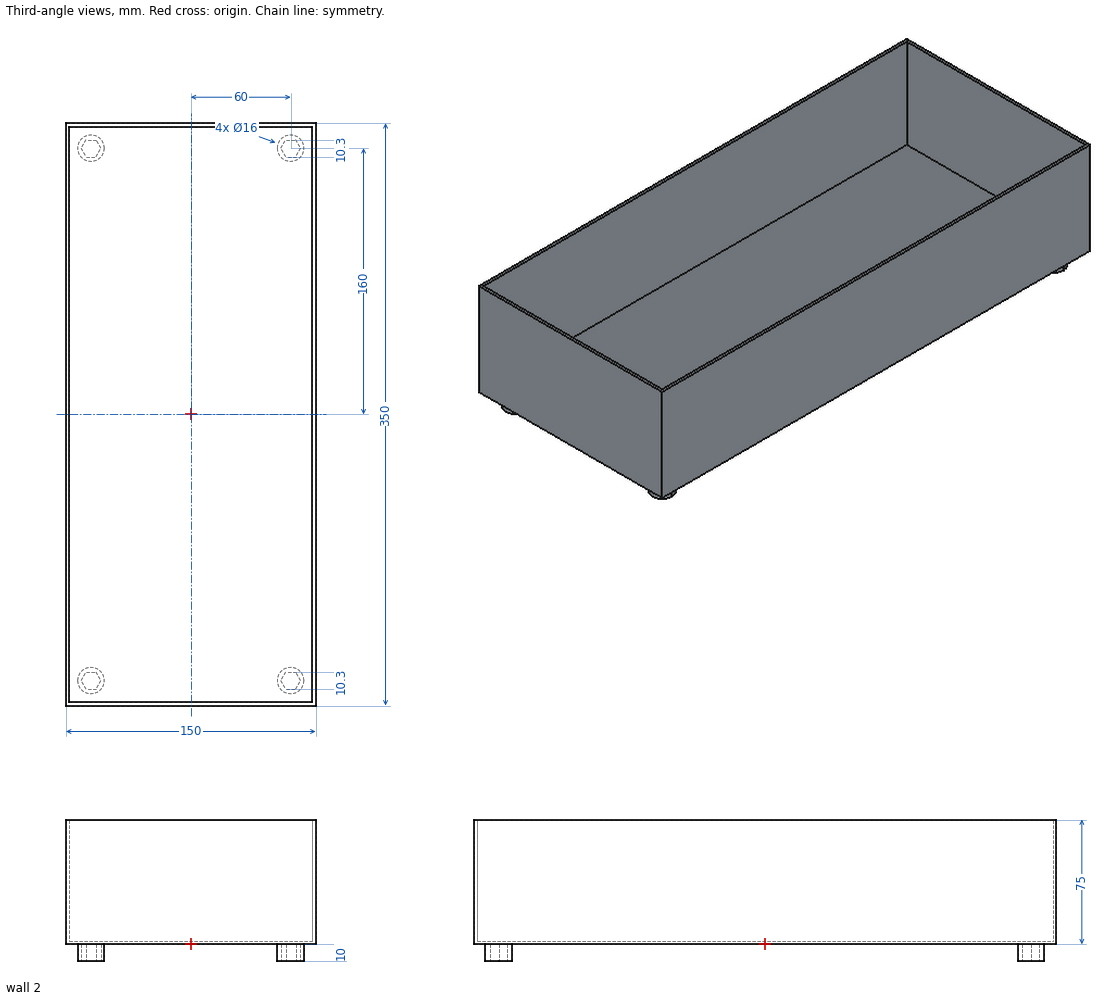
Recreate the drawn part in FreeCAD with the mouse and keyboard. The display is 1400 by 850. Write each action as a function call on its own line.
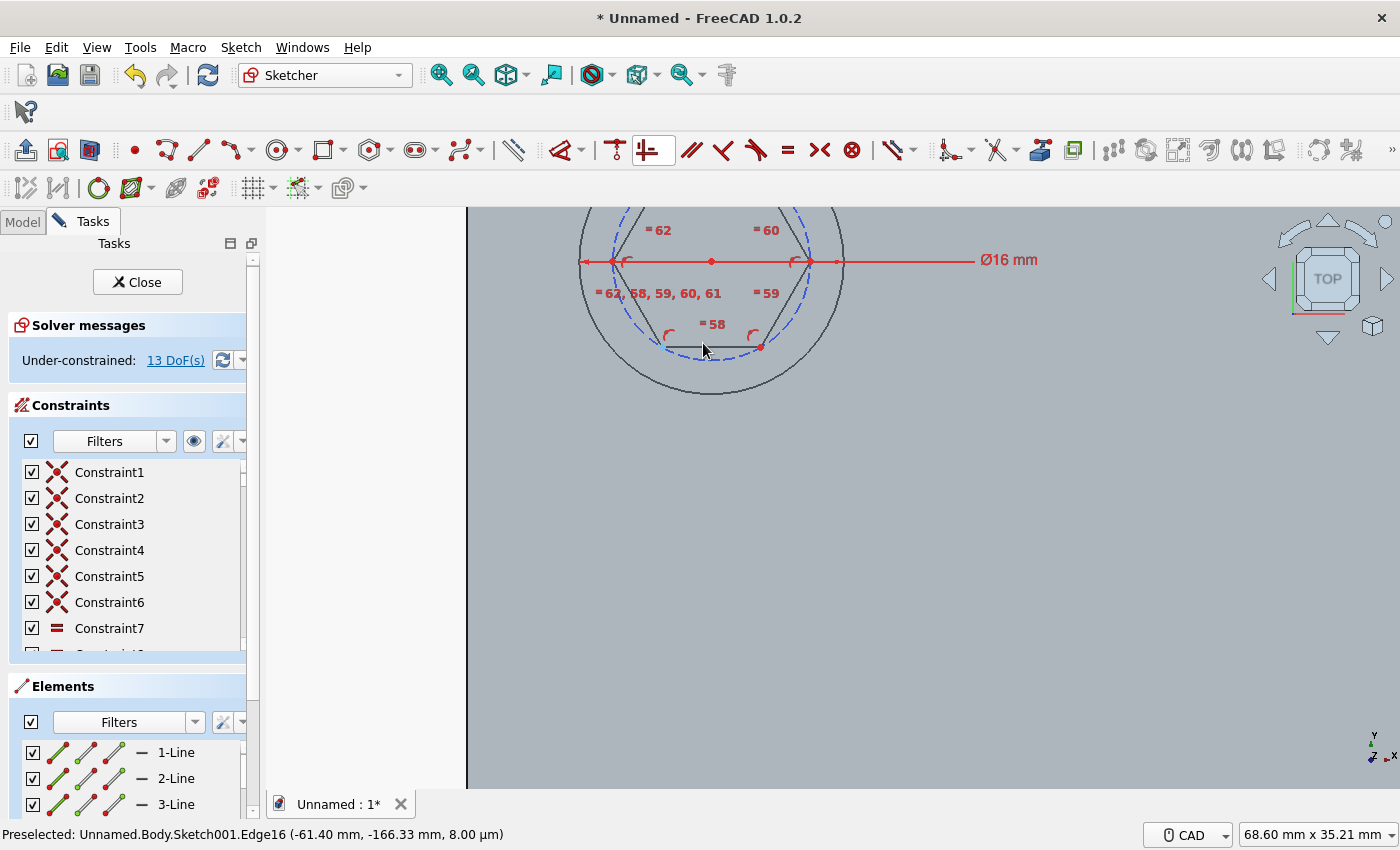
click(692, 347)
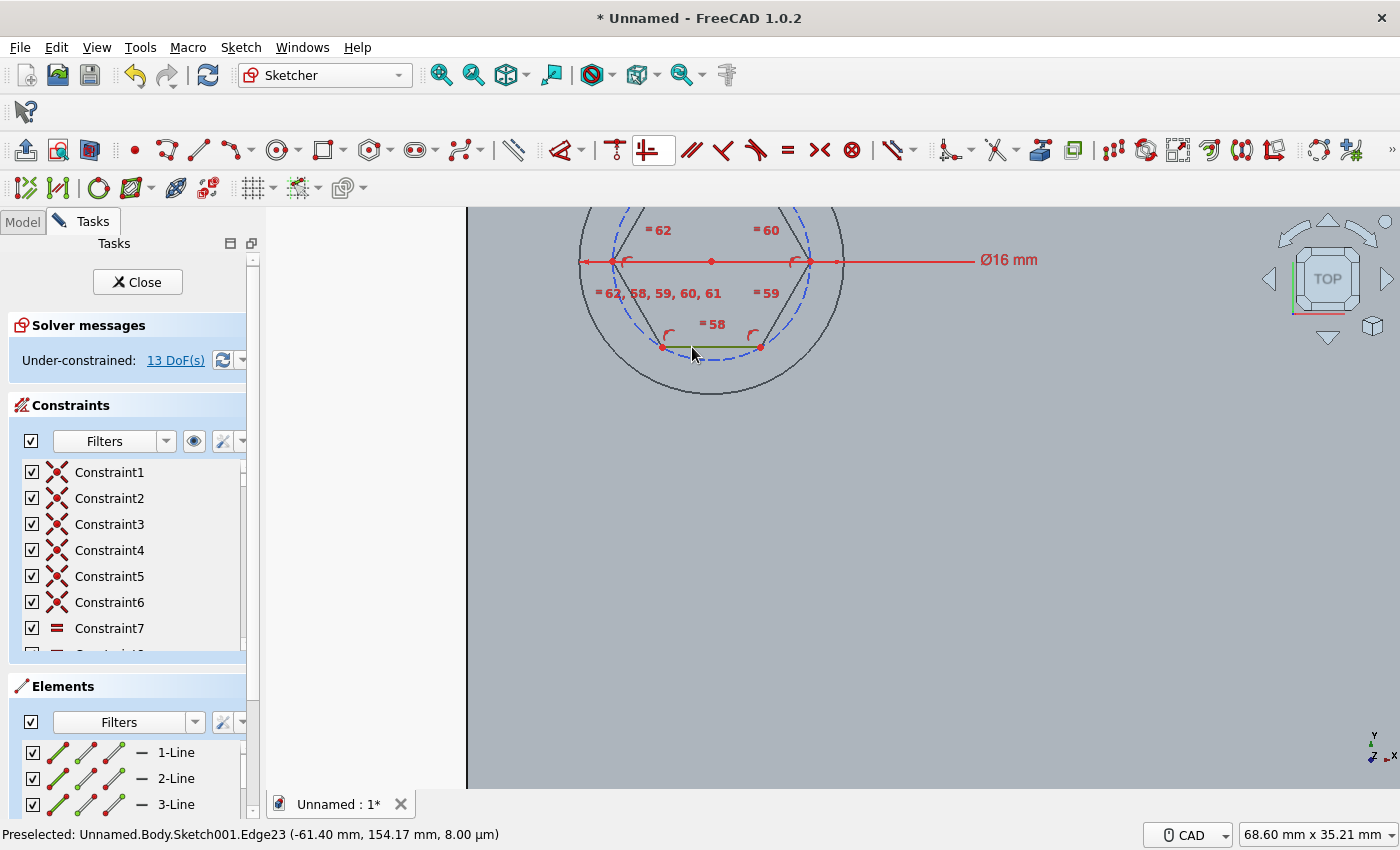
click(670, 150)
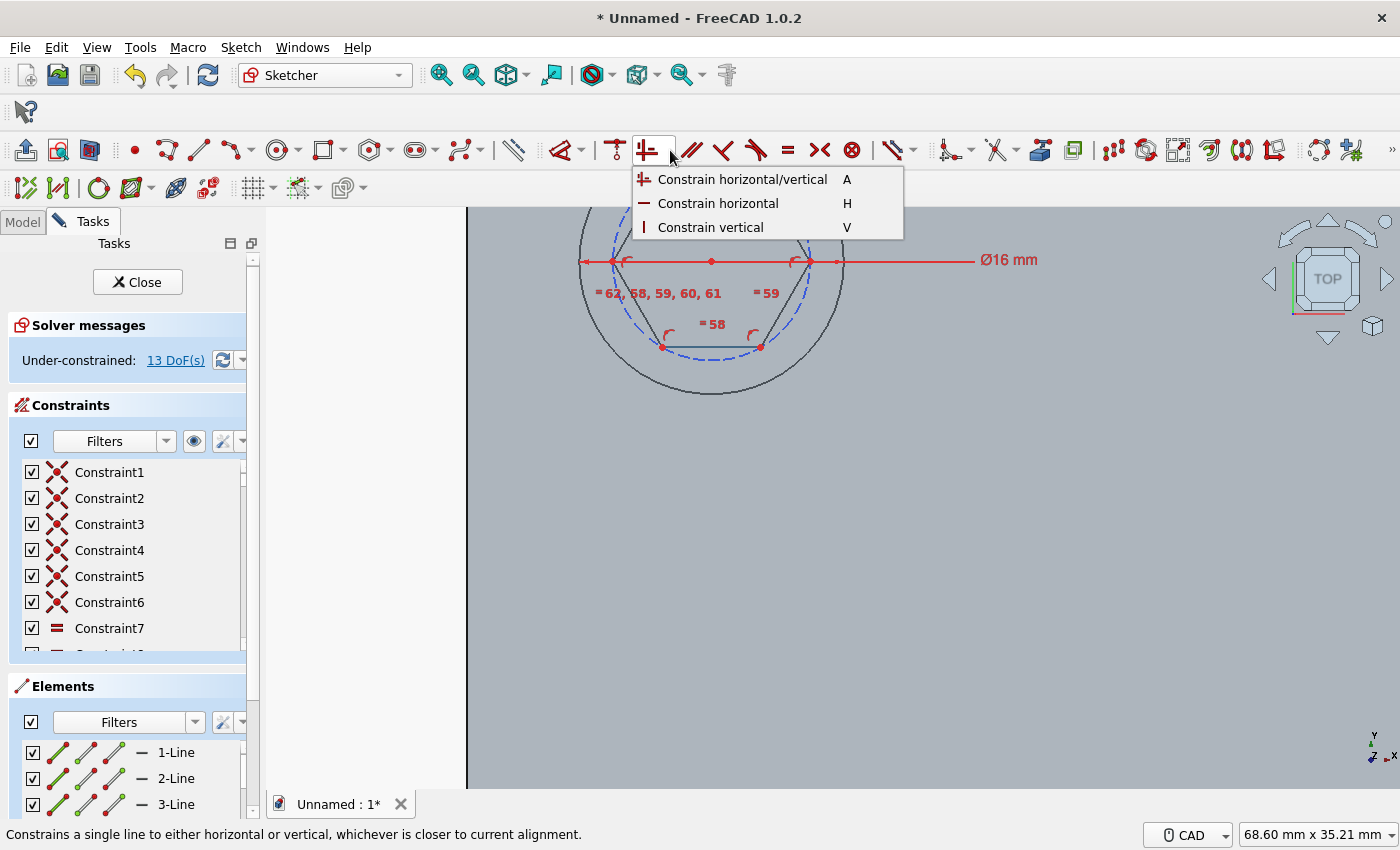
click(768, 203)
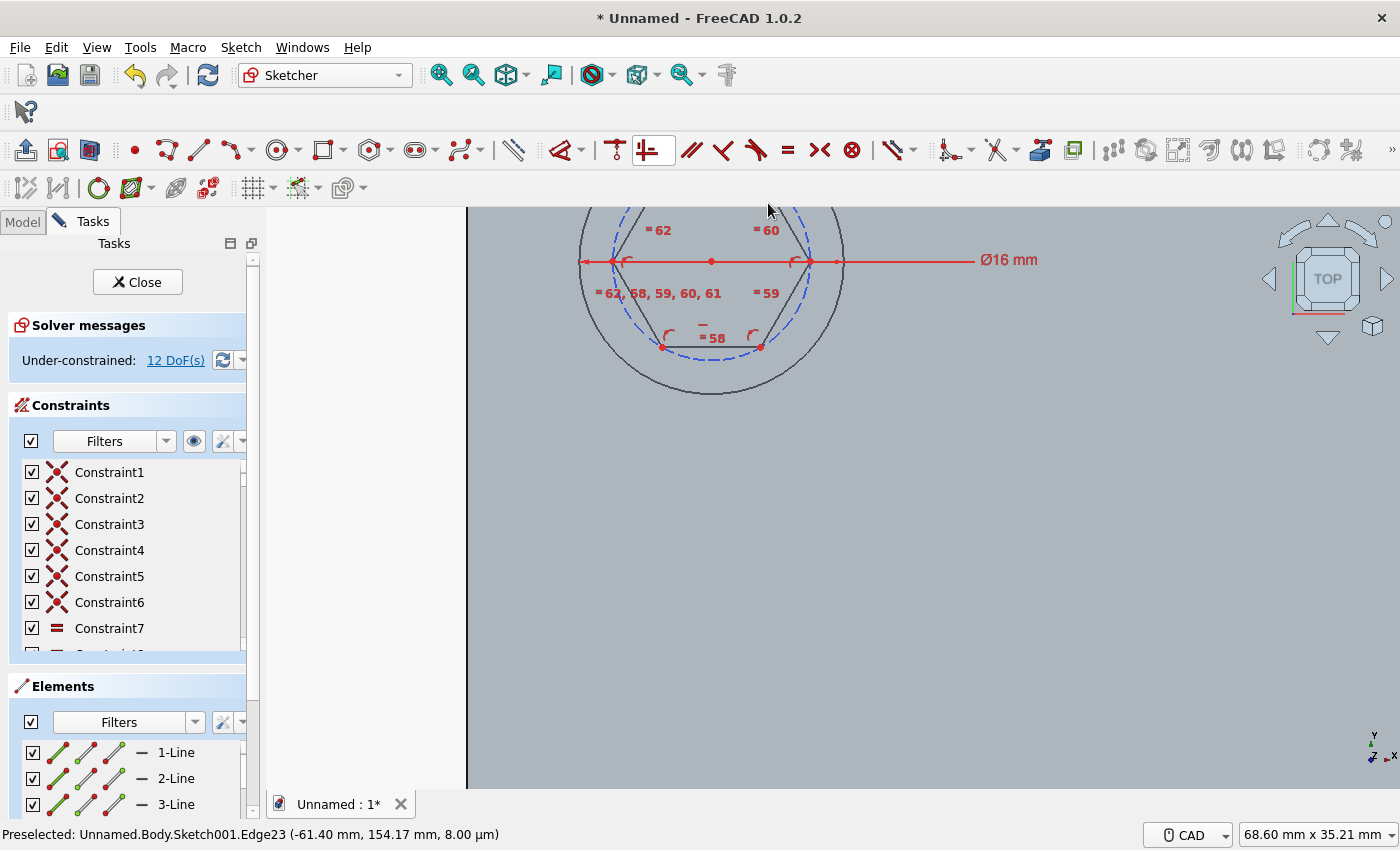
scroll(703, 343, down, 14)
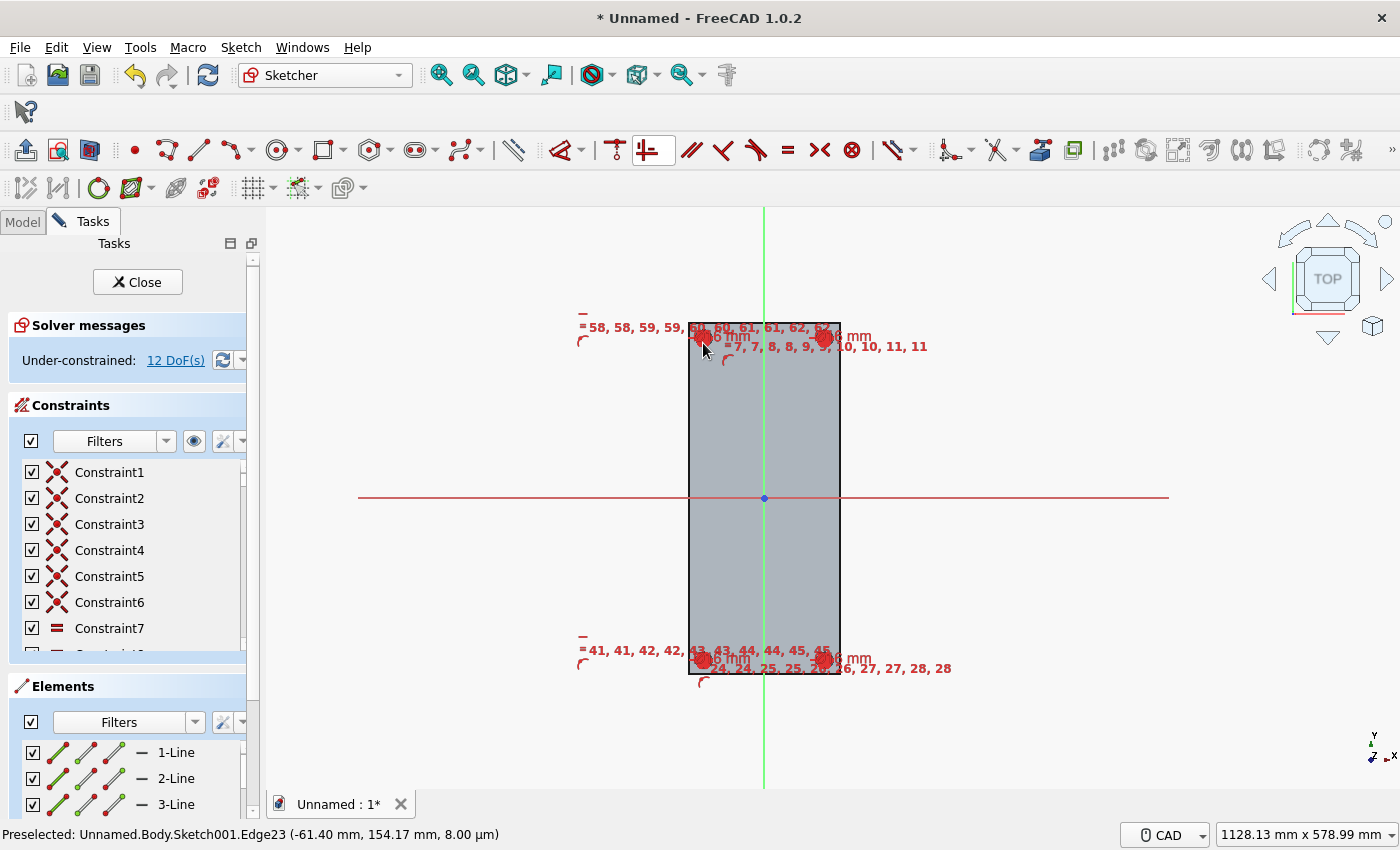
scroll(825, 338, up, 4)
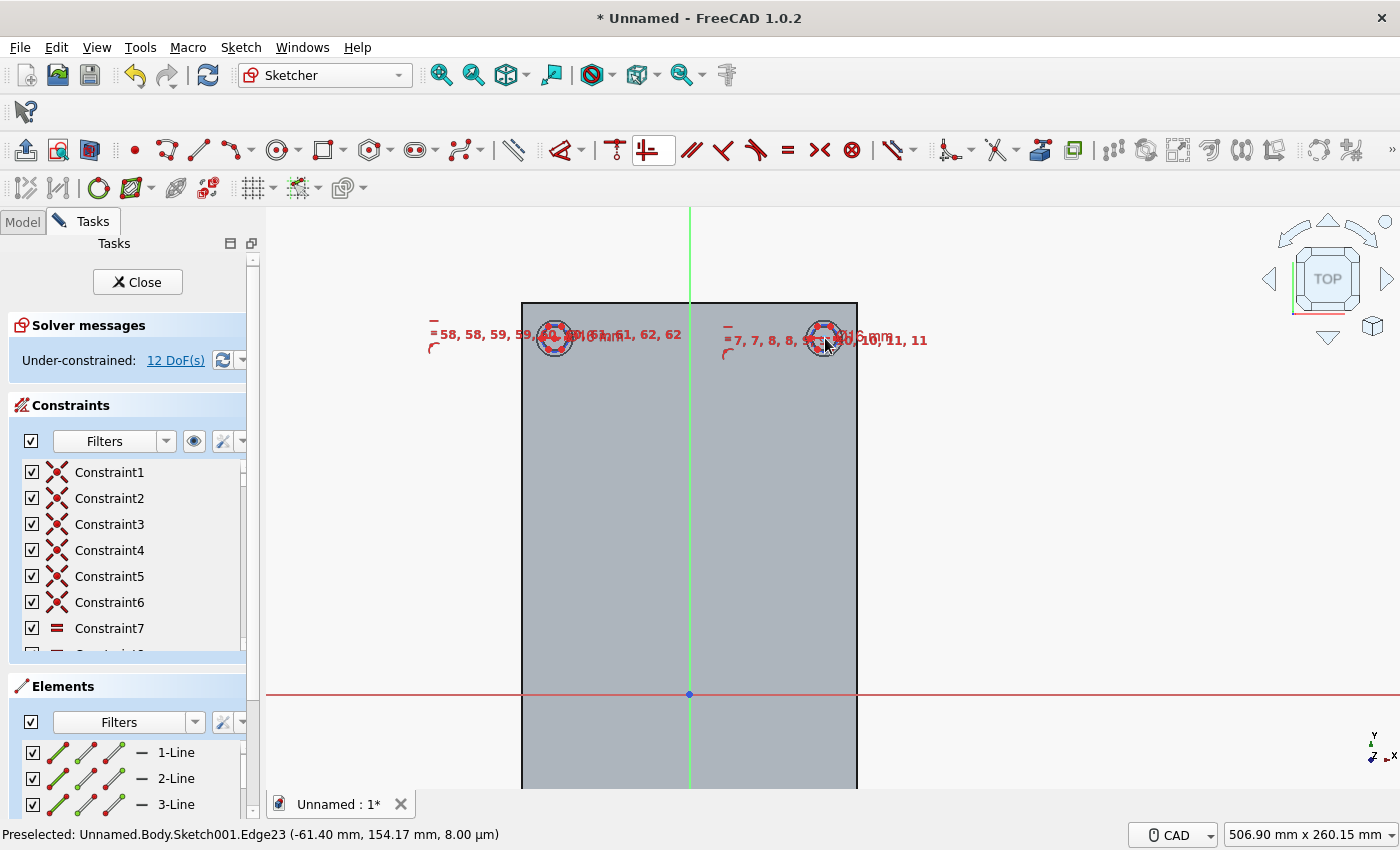
click(824, 338)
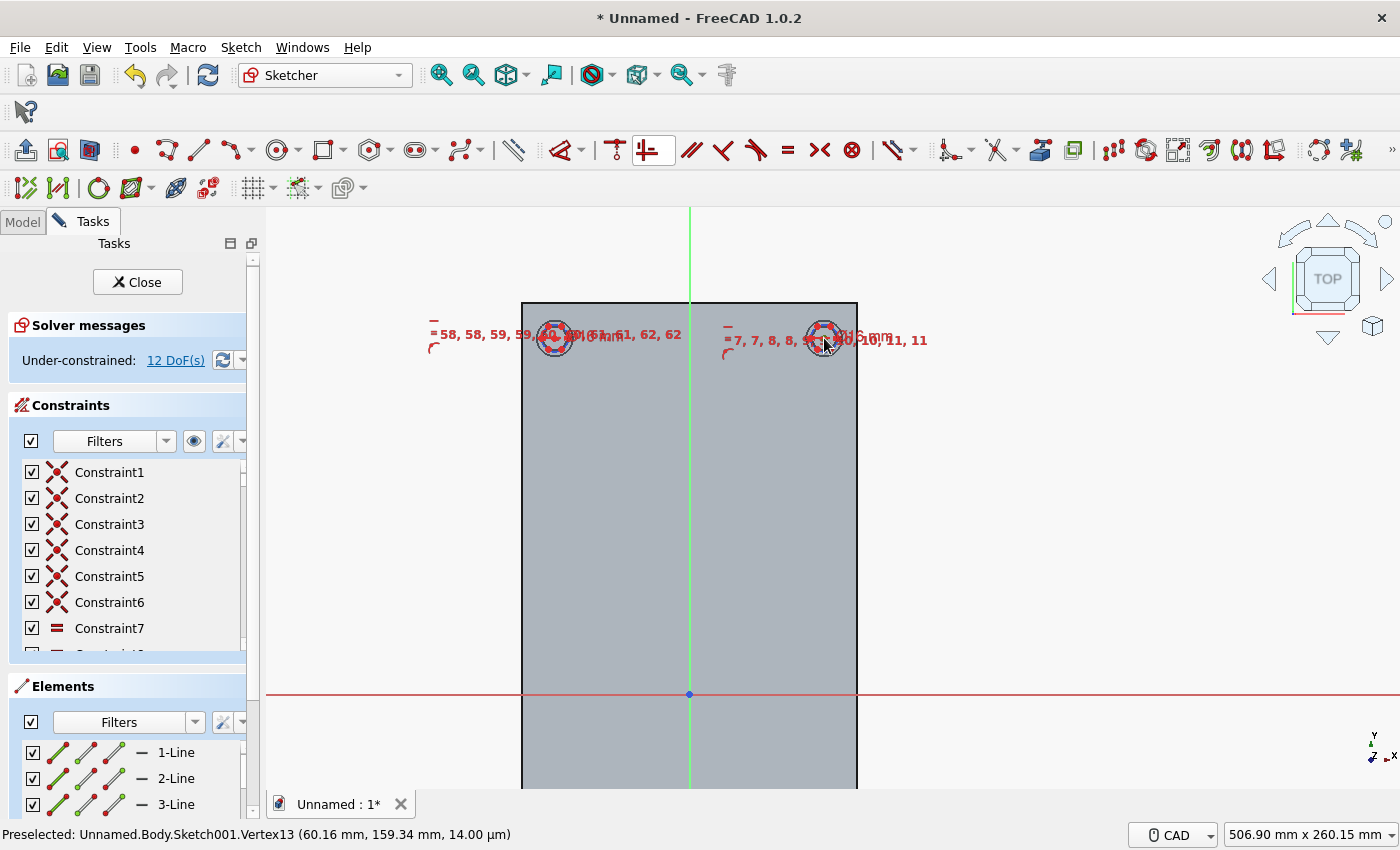
scroll(826, 337, down, 4)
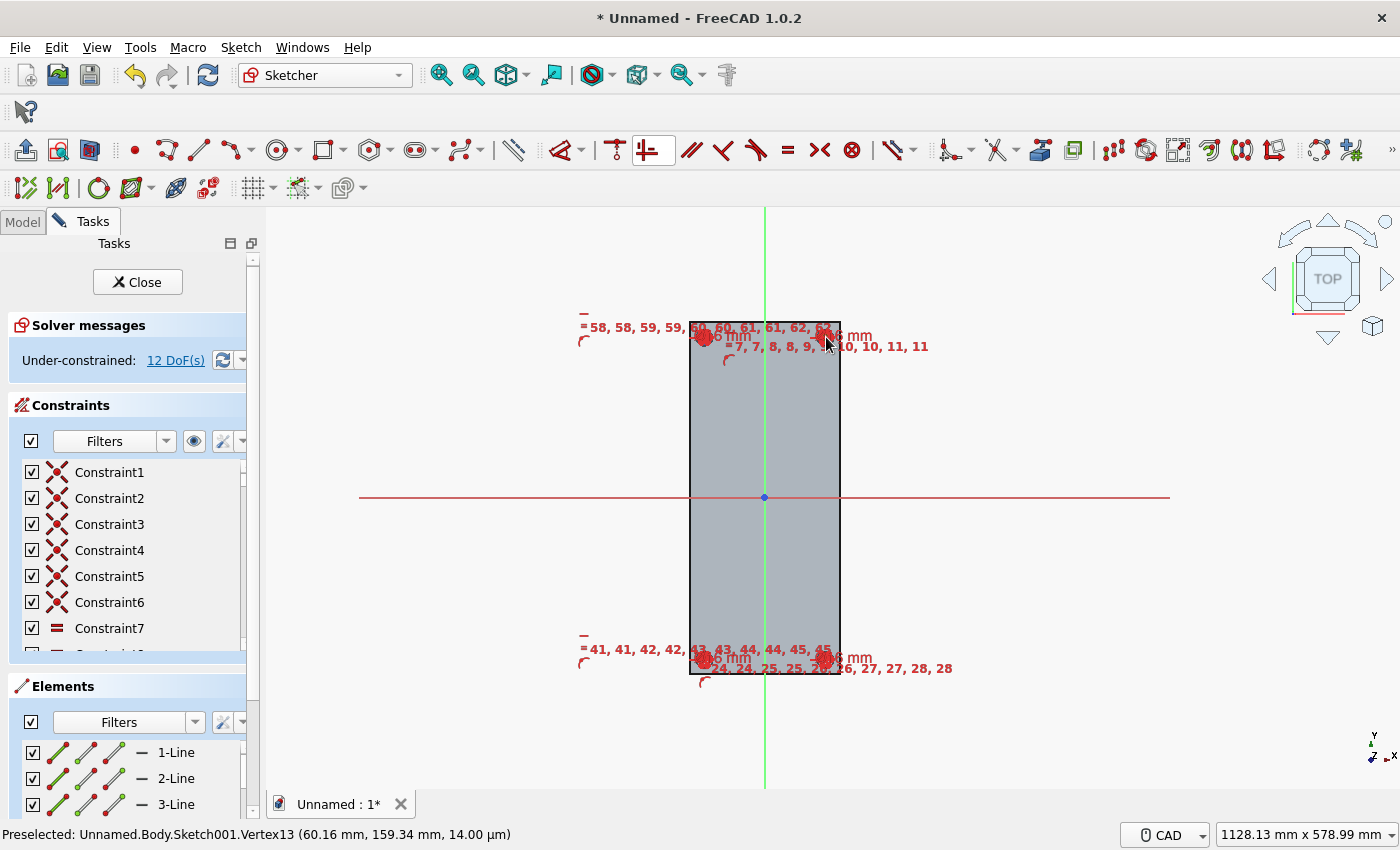
scroll(825, 660, up, 4)